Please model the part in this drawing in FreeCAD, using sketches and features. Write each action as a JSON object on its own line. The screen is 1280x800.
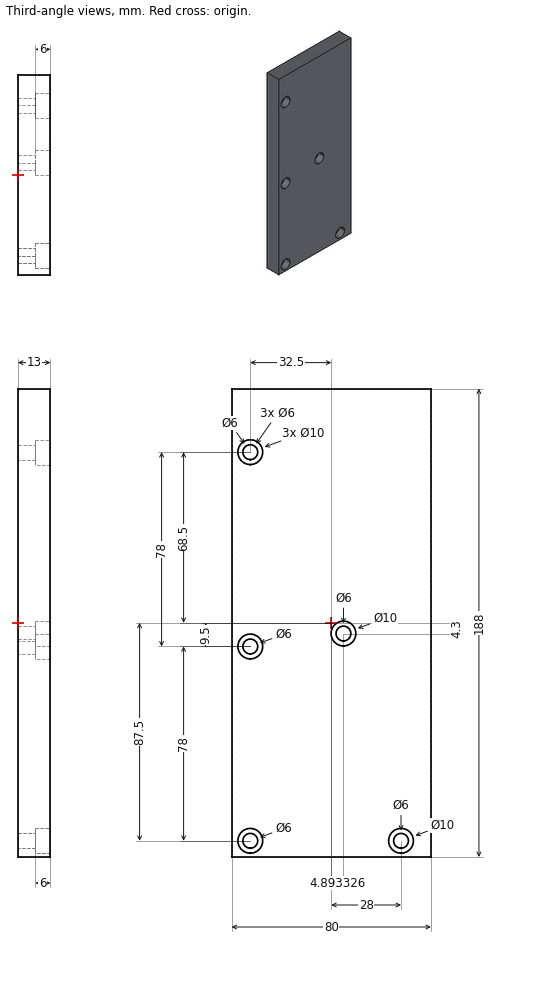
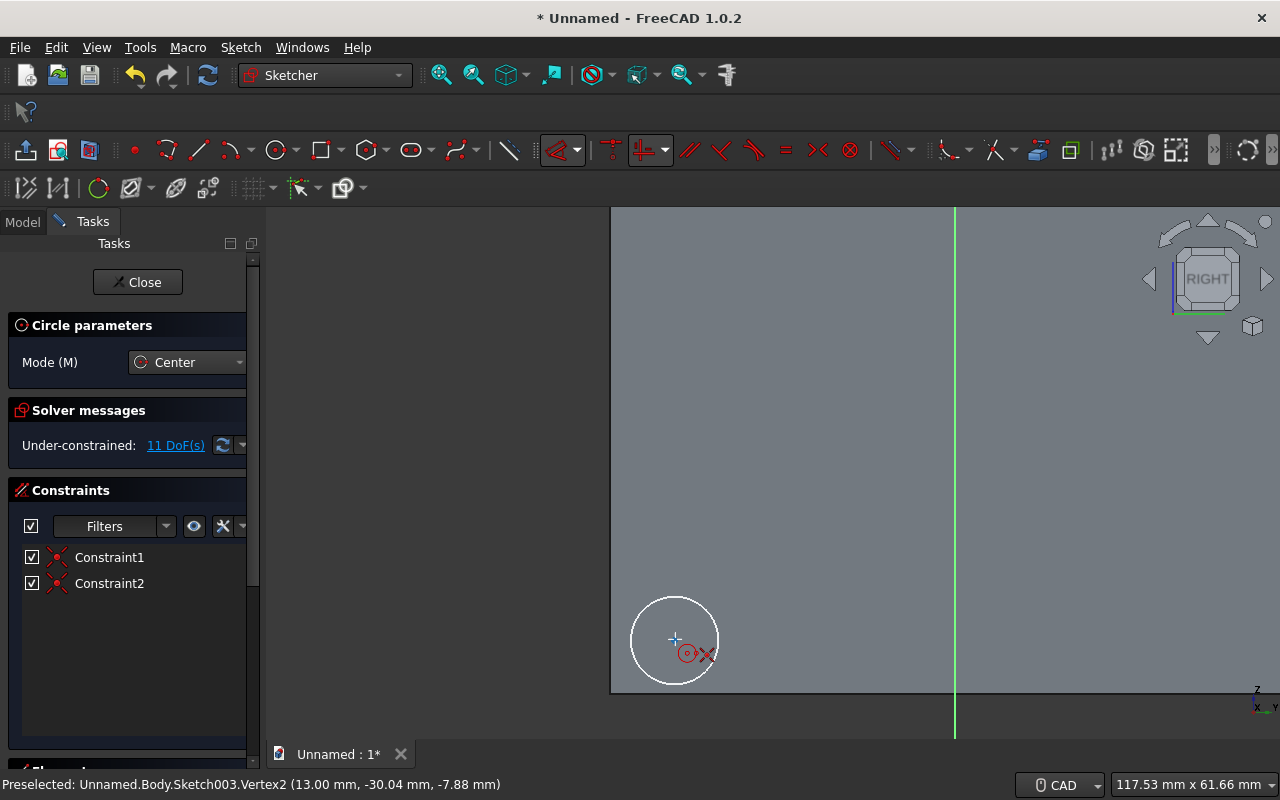
{"action": "left_click", "coordinate": [675, 641]}
{"action": "left_click", "coordinate": [693, 620]}
{"action": "key", "text": "Escape"}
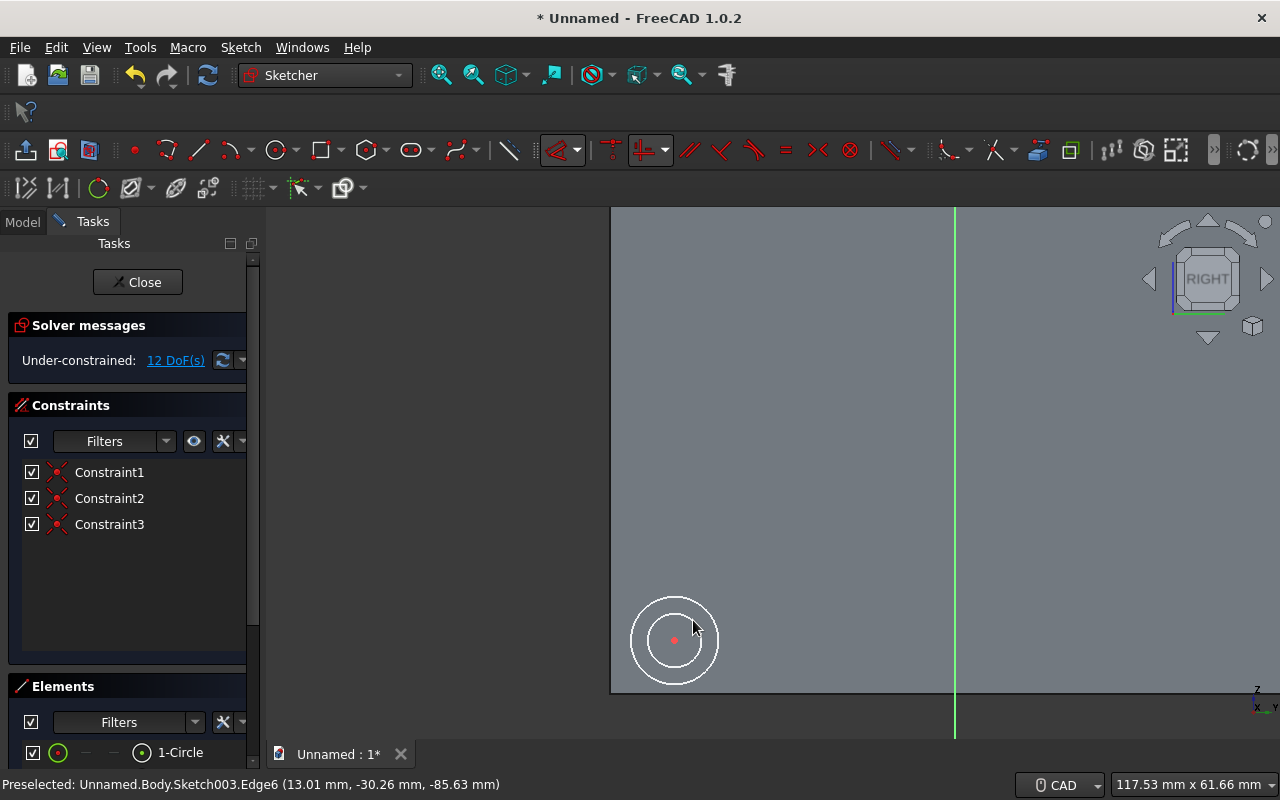
{"action": "scroll", "coordinate": [675, 639], "scroll_direction": "down", "scroll_amount": 7}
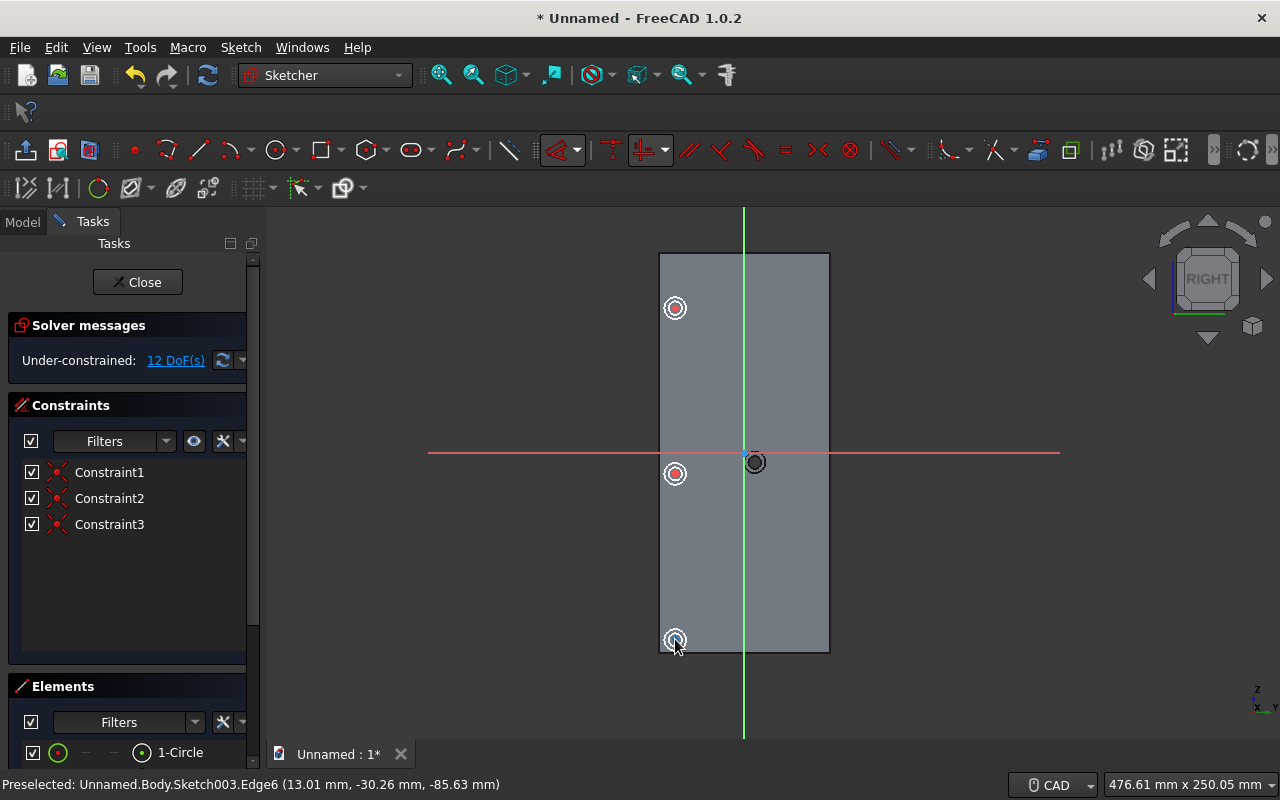
{"action": "scroll", "coordinate": [683, 300], "scroll_direction": "up", "scroll_amount": 7}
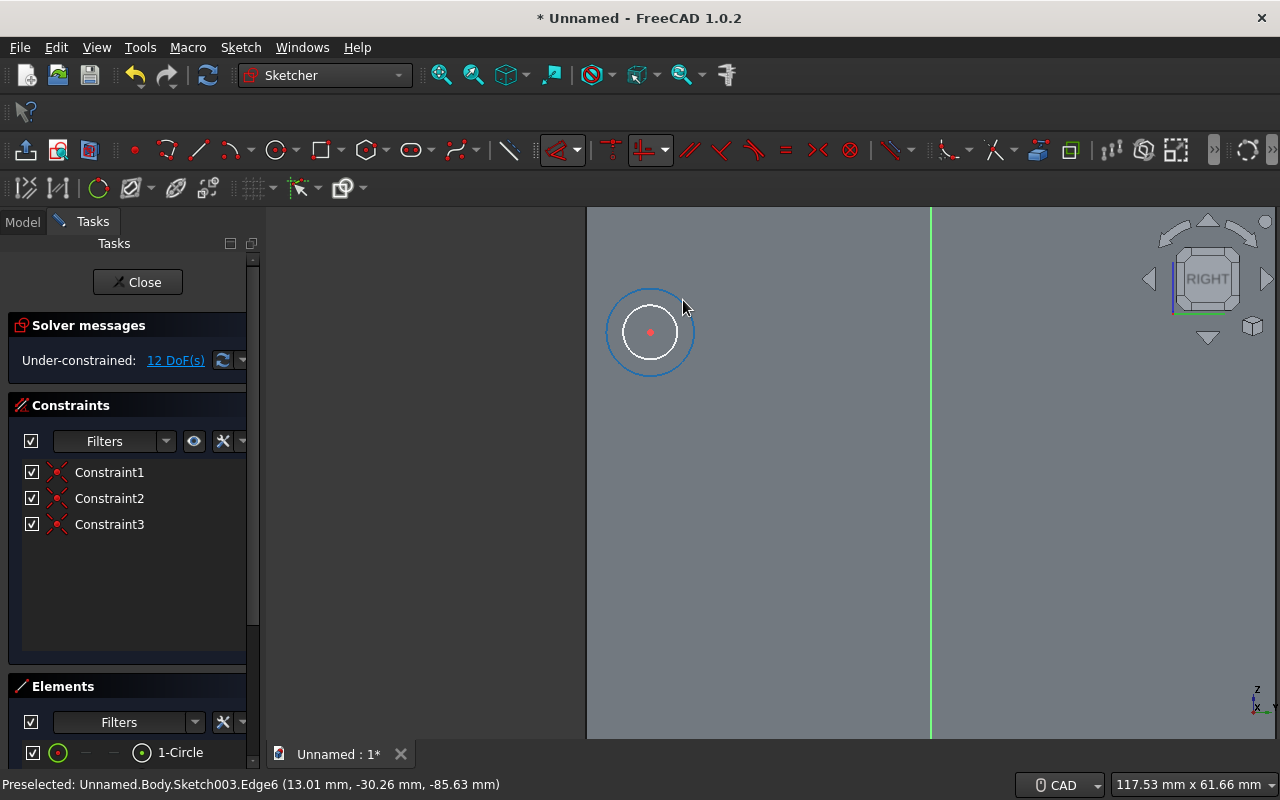
{"action": "left_click", "coordinate": [681, 301]}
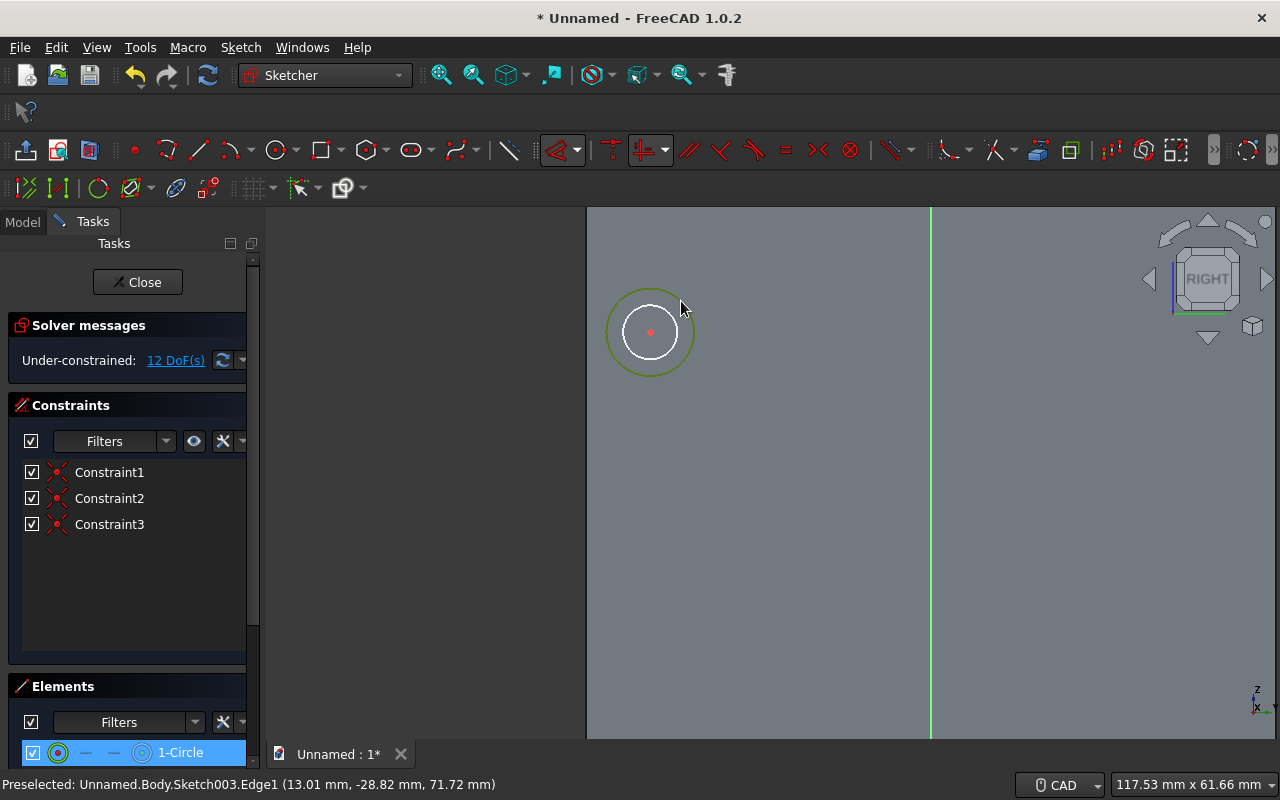
{"action": "scroll", "coordinate": [683, 299], "scroll_direction": "down", "scroll_amount": 7}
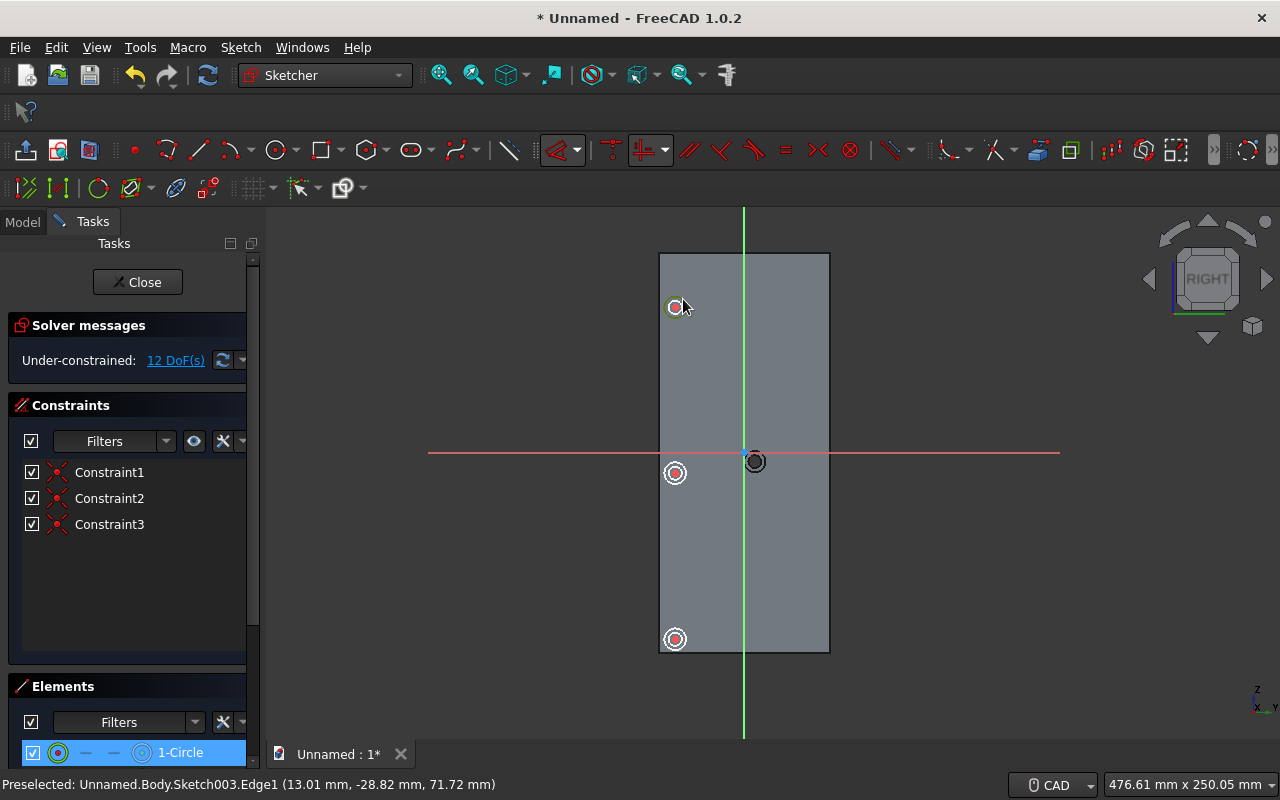
{"action": "scroll", "coordinate": [683, 465], "scroll_direction": "up", "scroll_amount": 6}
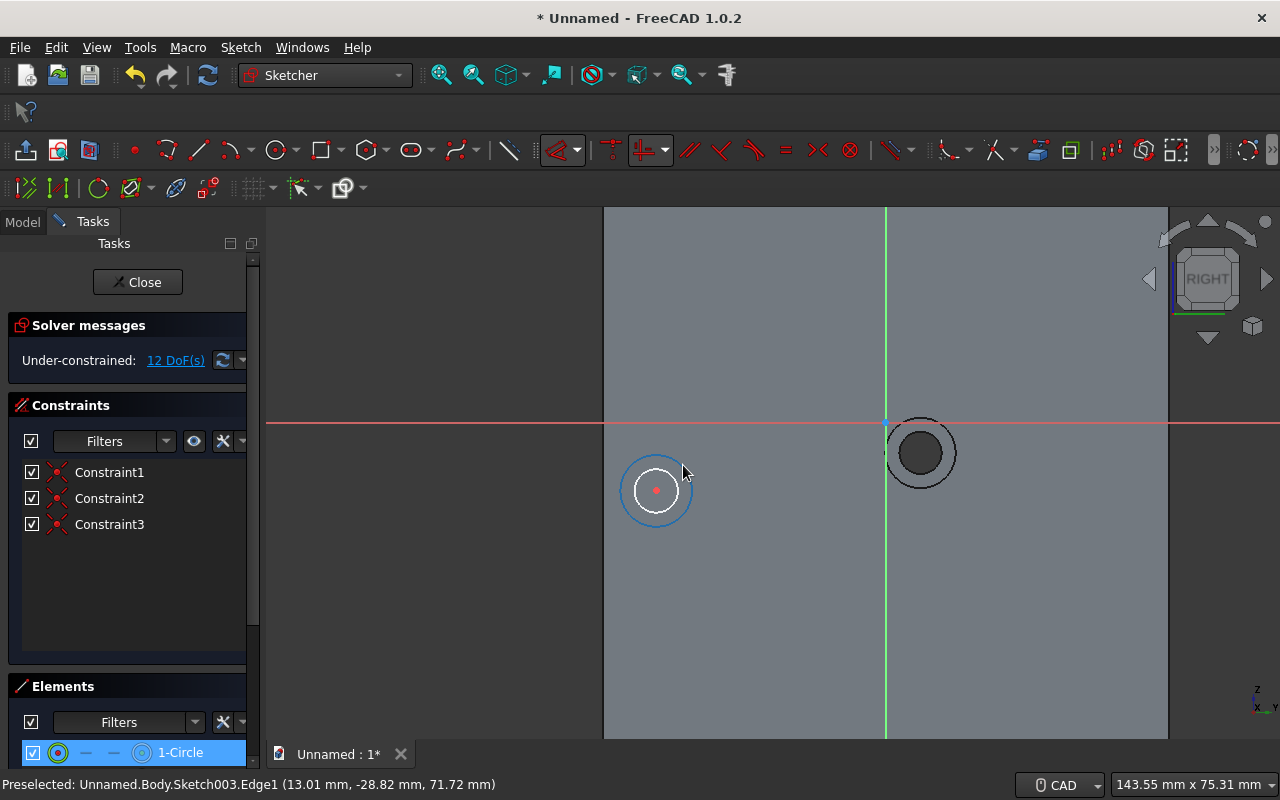
{"action": "left_click", "coordinate": [682, 465]}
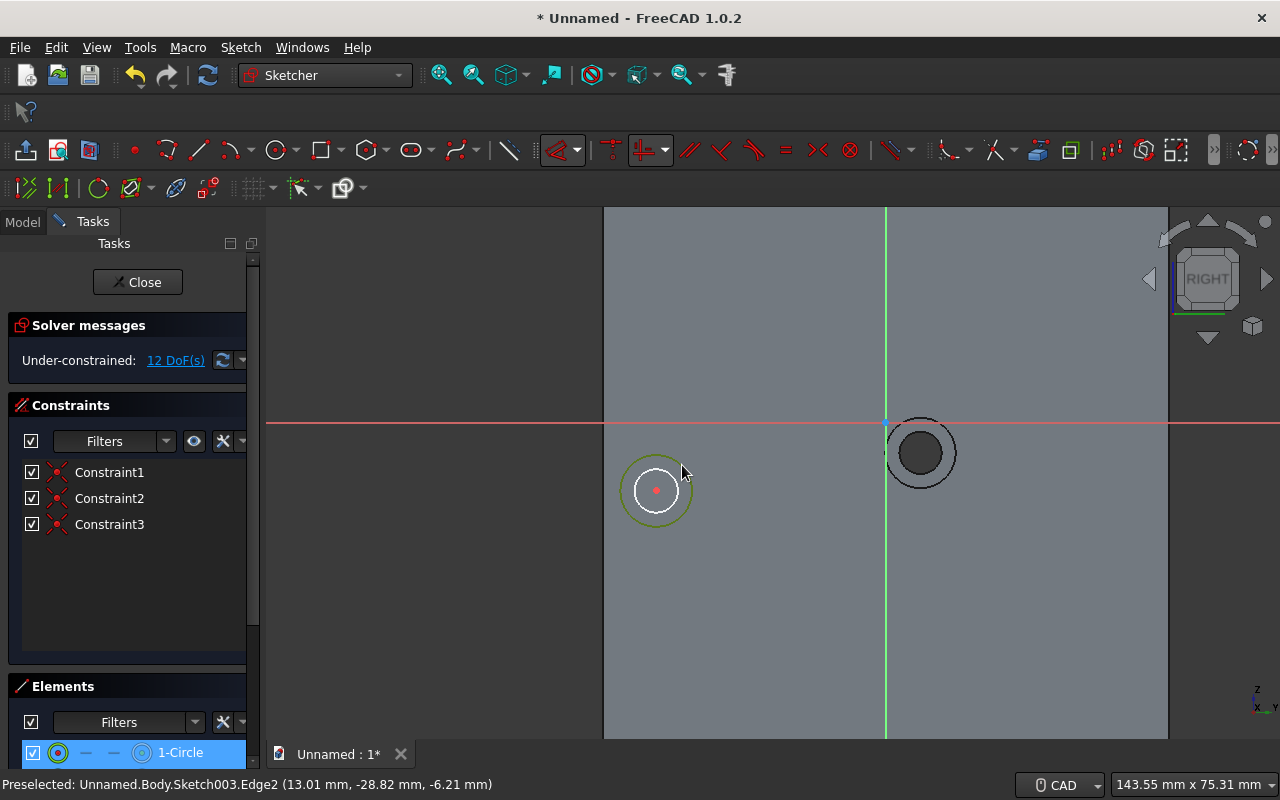
{"action": "scroll", "coordinate": [683, 466], "scroll_direction": "down", "scroll_amount": 6}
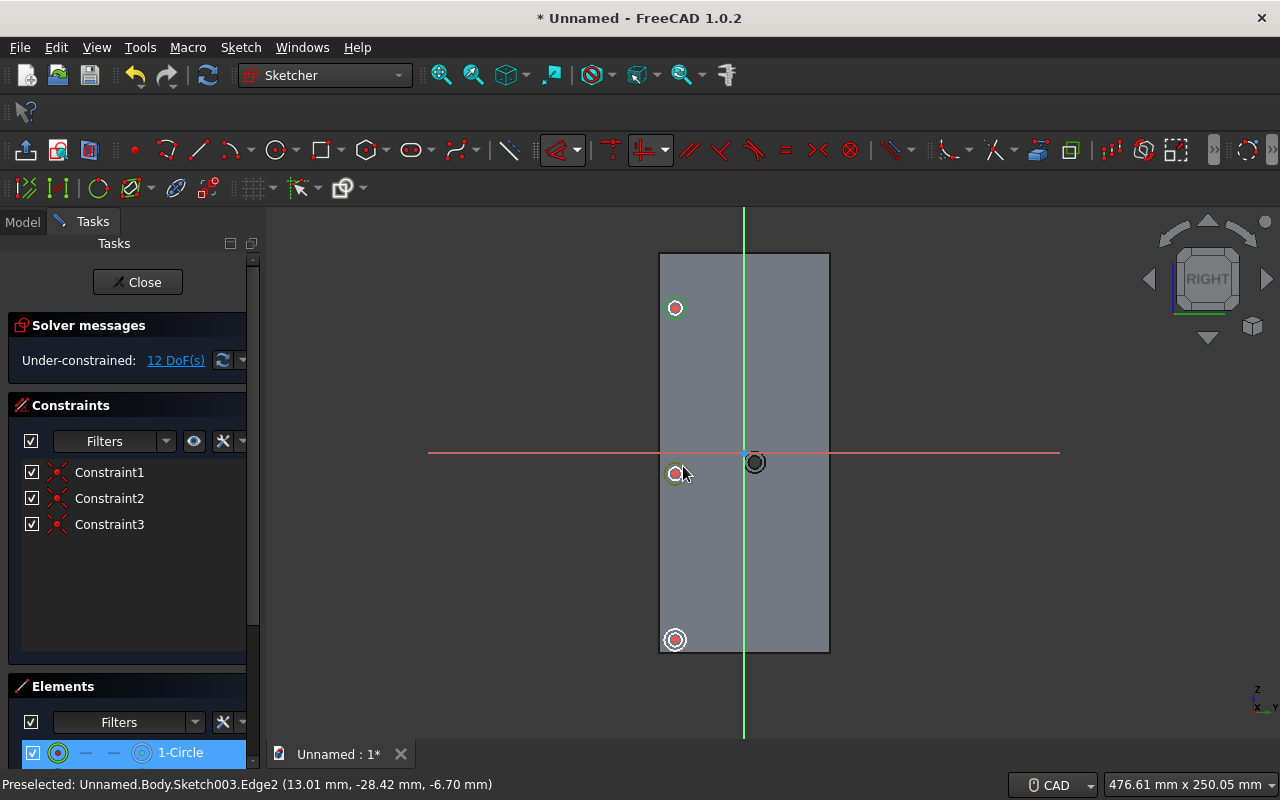
{"action": "scroll", "coordinate": [683, 632], "scroll_direction": "up", "scroll_amount": 6}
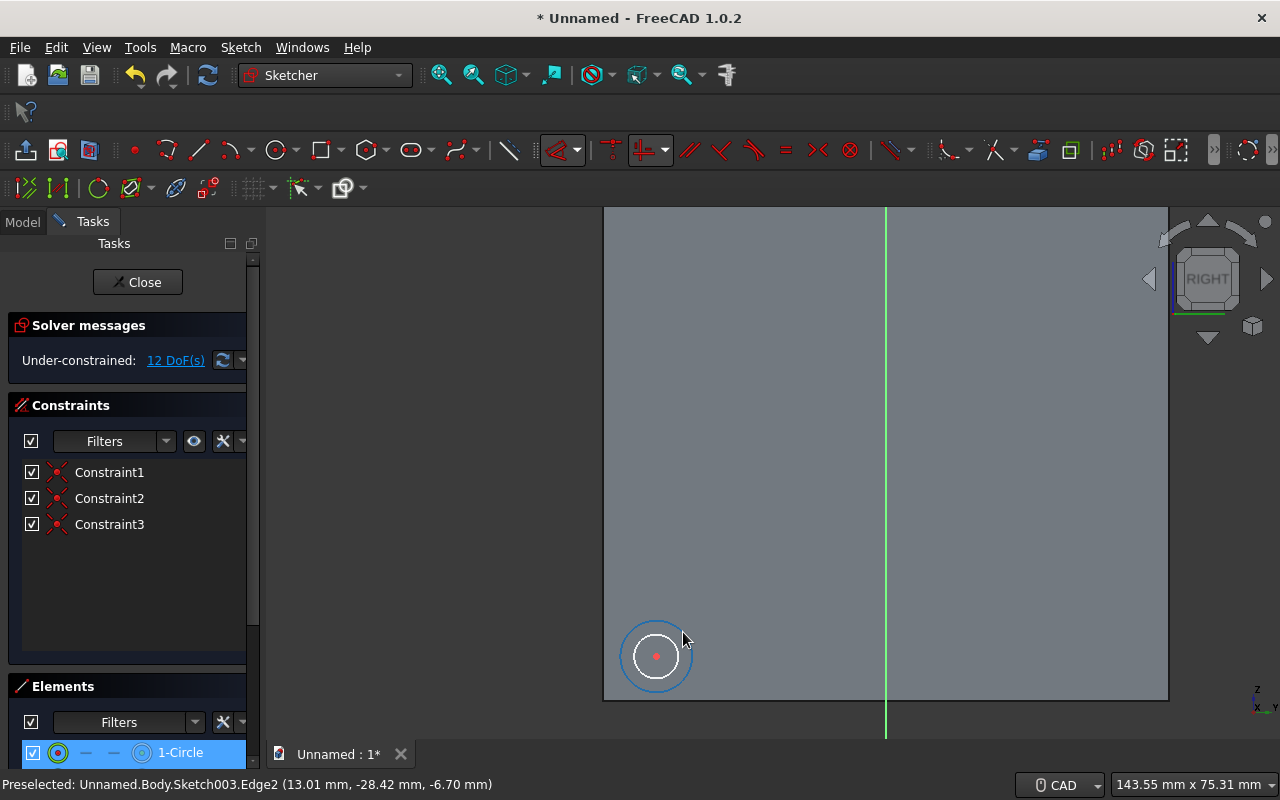
{"action": "left_click", "coordinate": [682, 631]}